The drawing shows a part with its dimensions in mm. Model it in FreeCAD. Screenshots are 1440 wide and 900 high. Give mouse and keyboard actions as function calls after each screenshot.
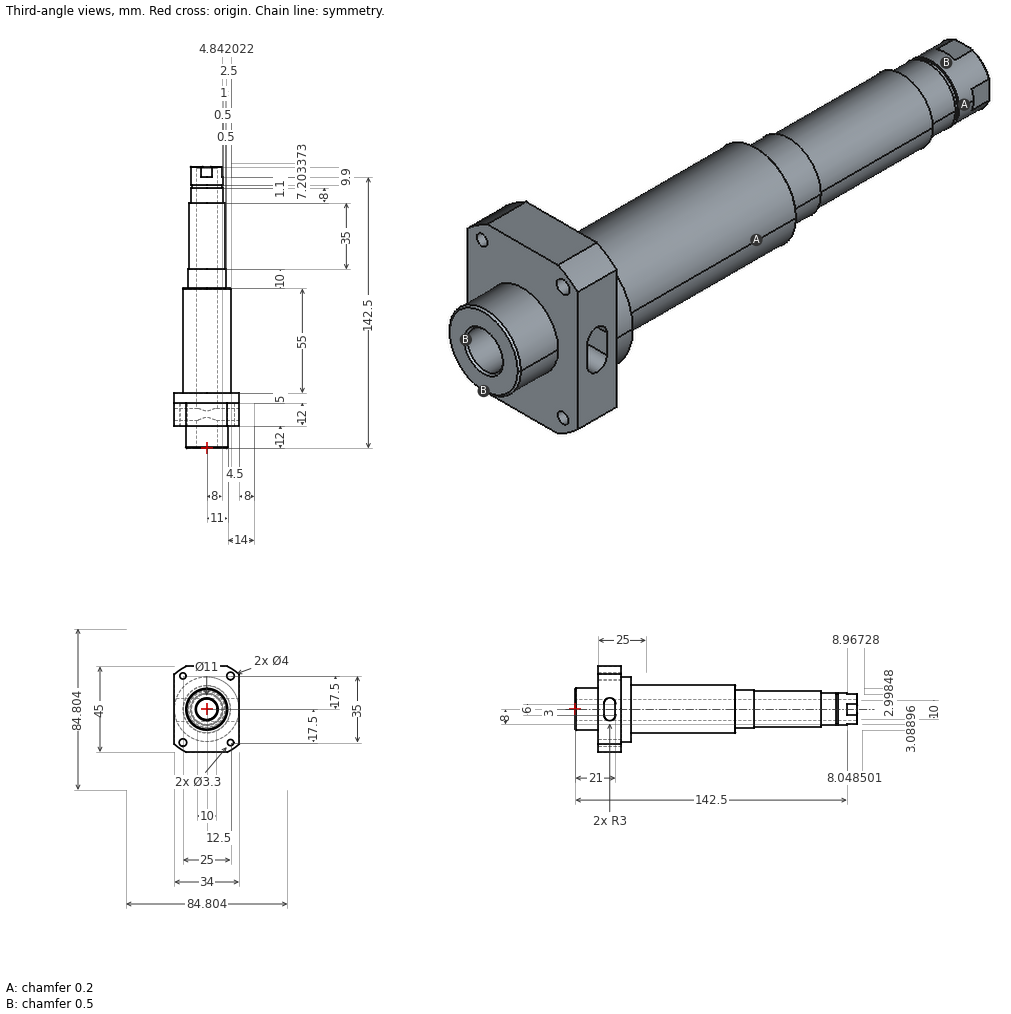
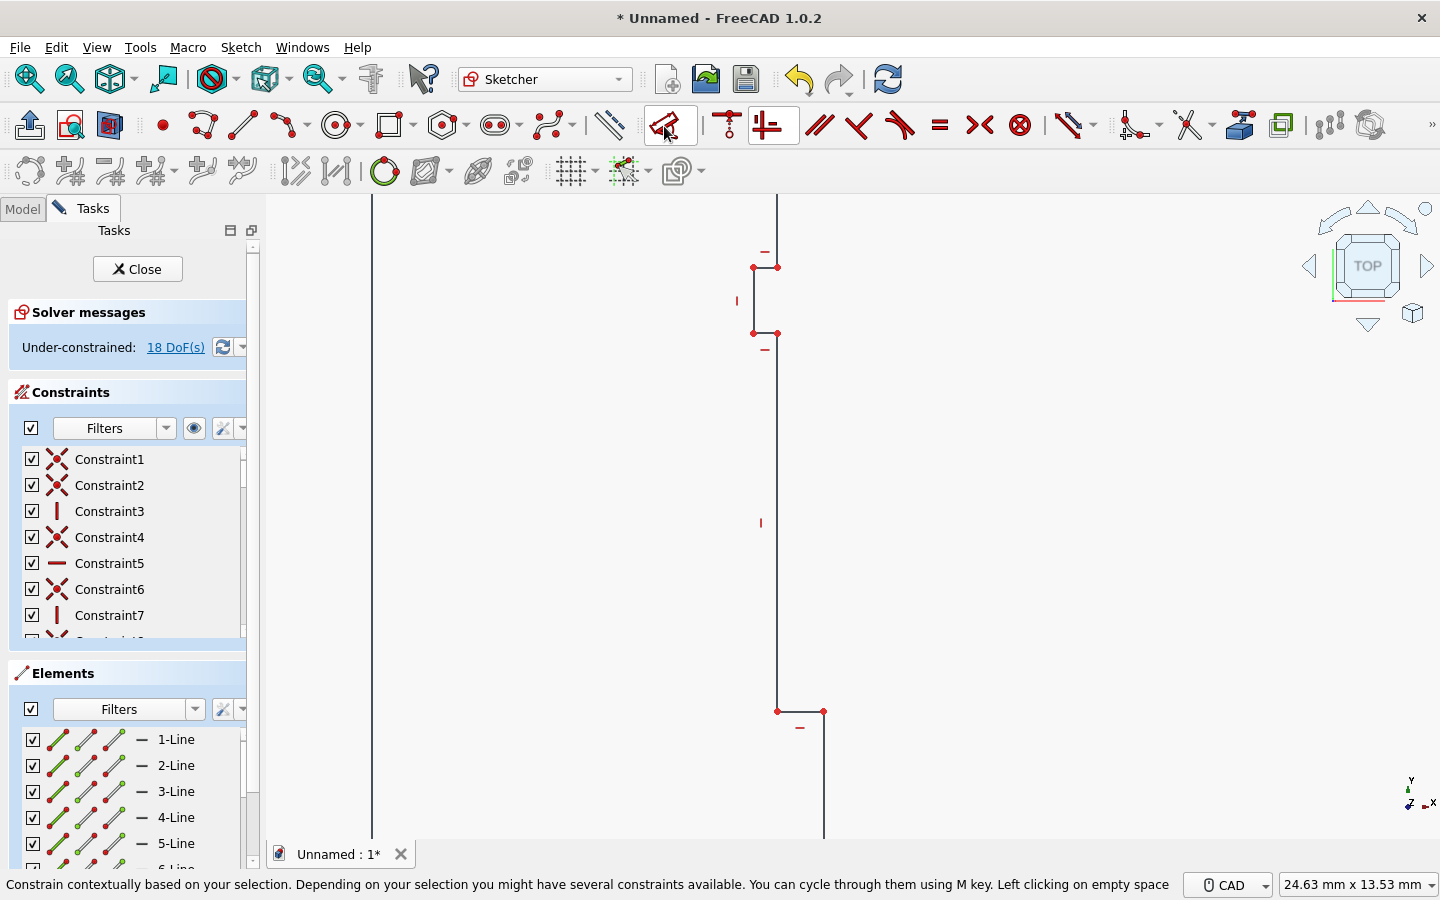
scroll(773, 335, down, 14)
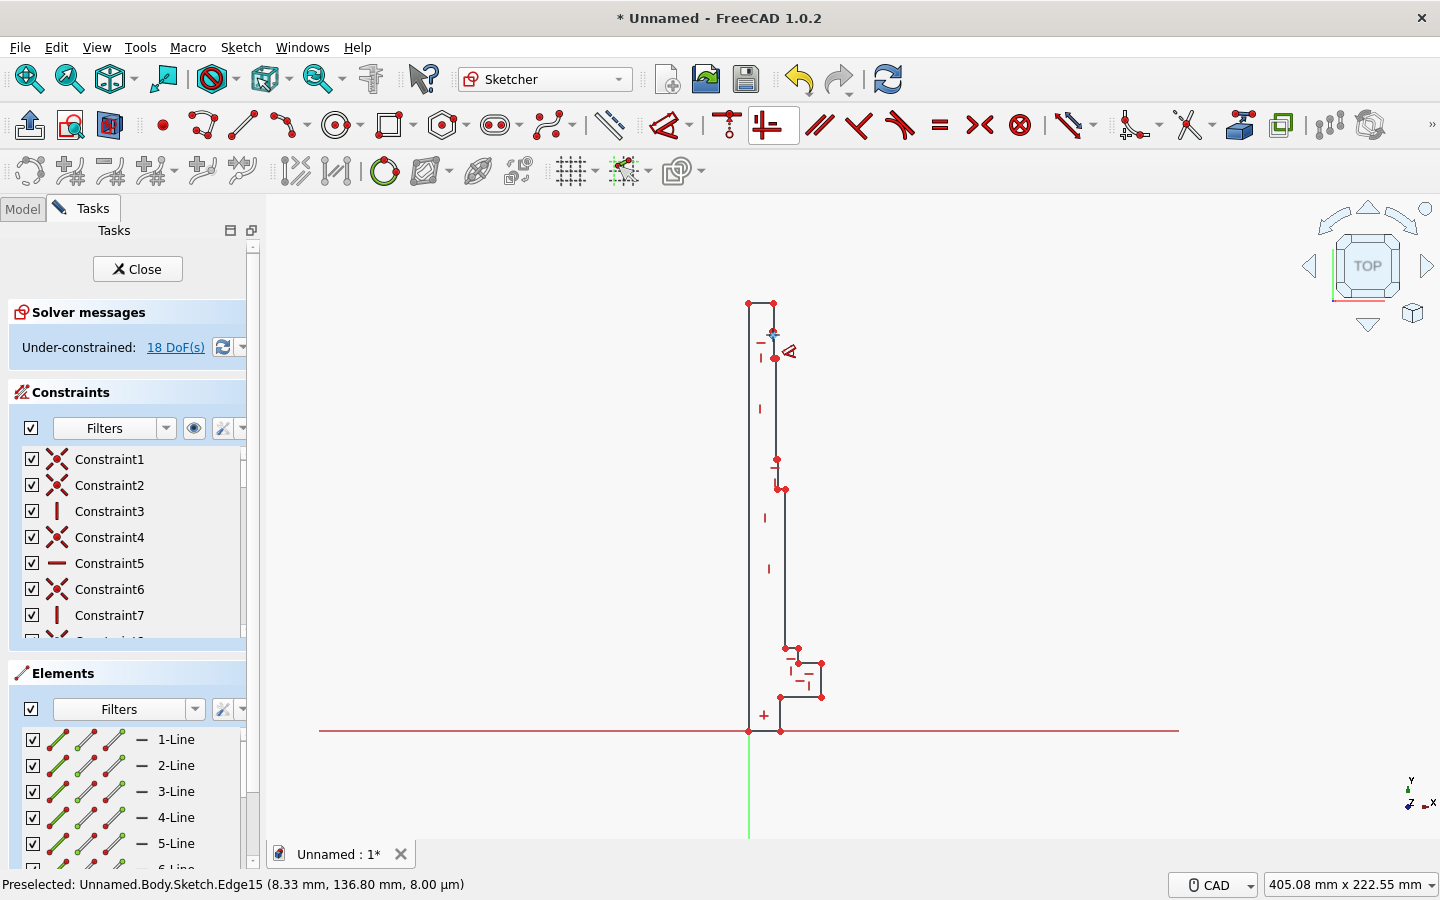
scroll(815, 663, up, 4)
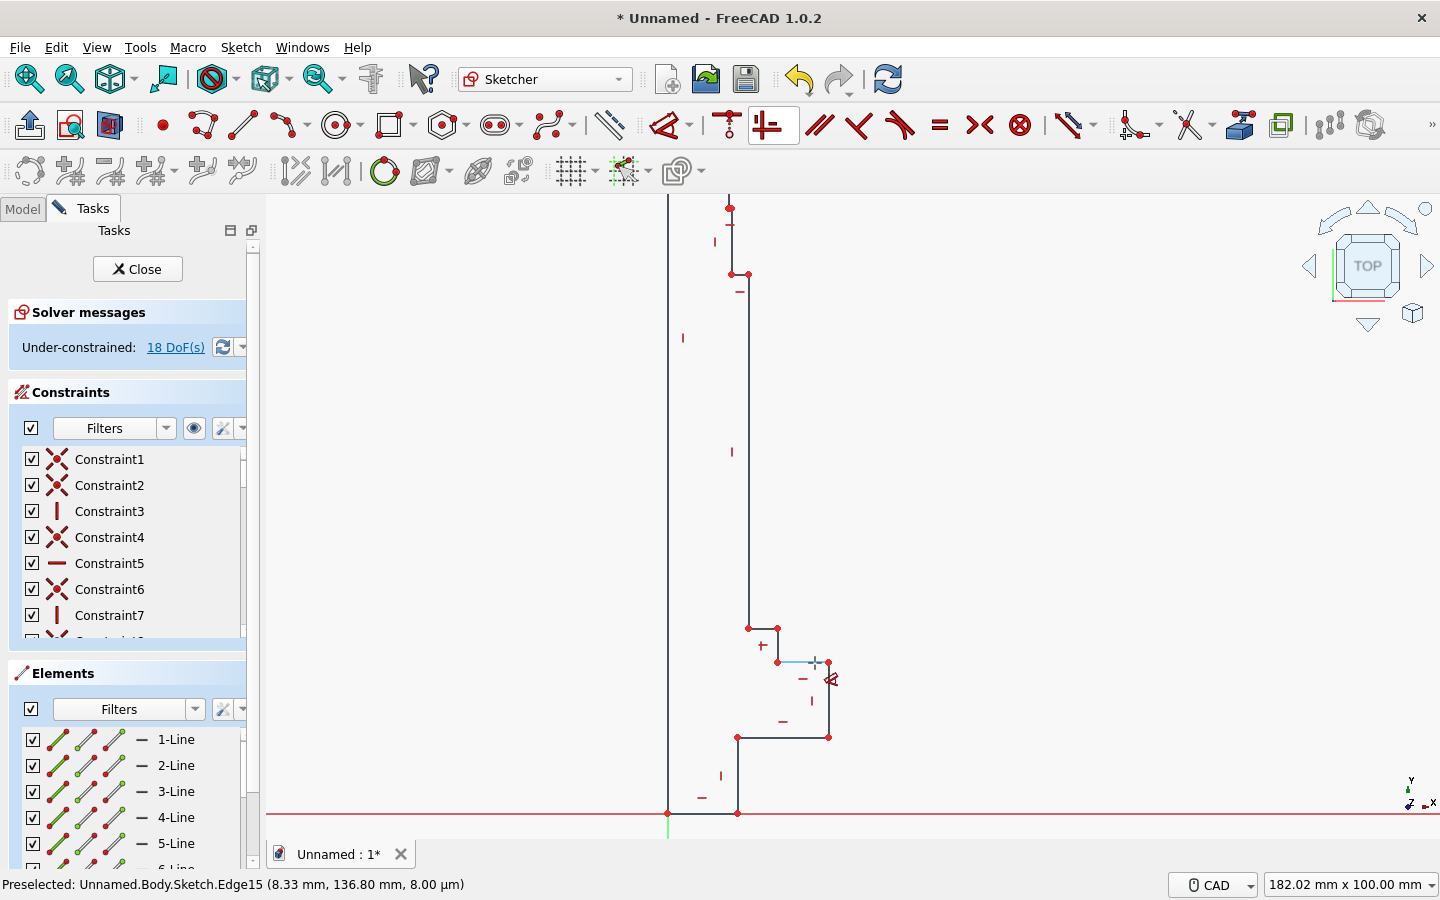
click(813, 662)
click(803, 696)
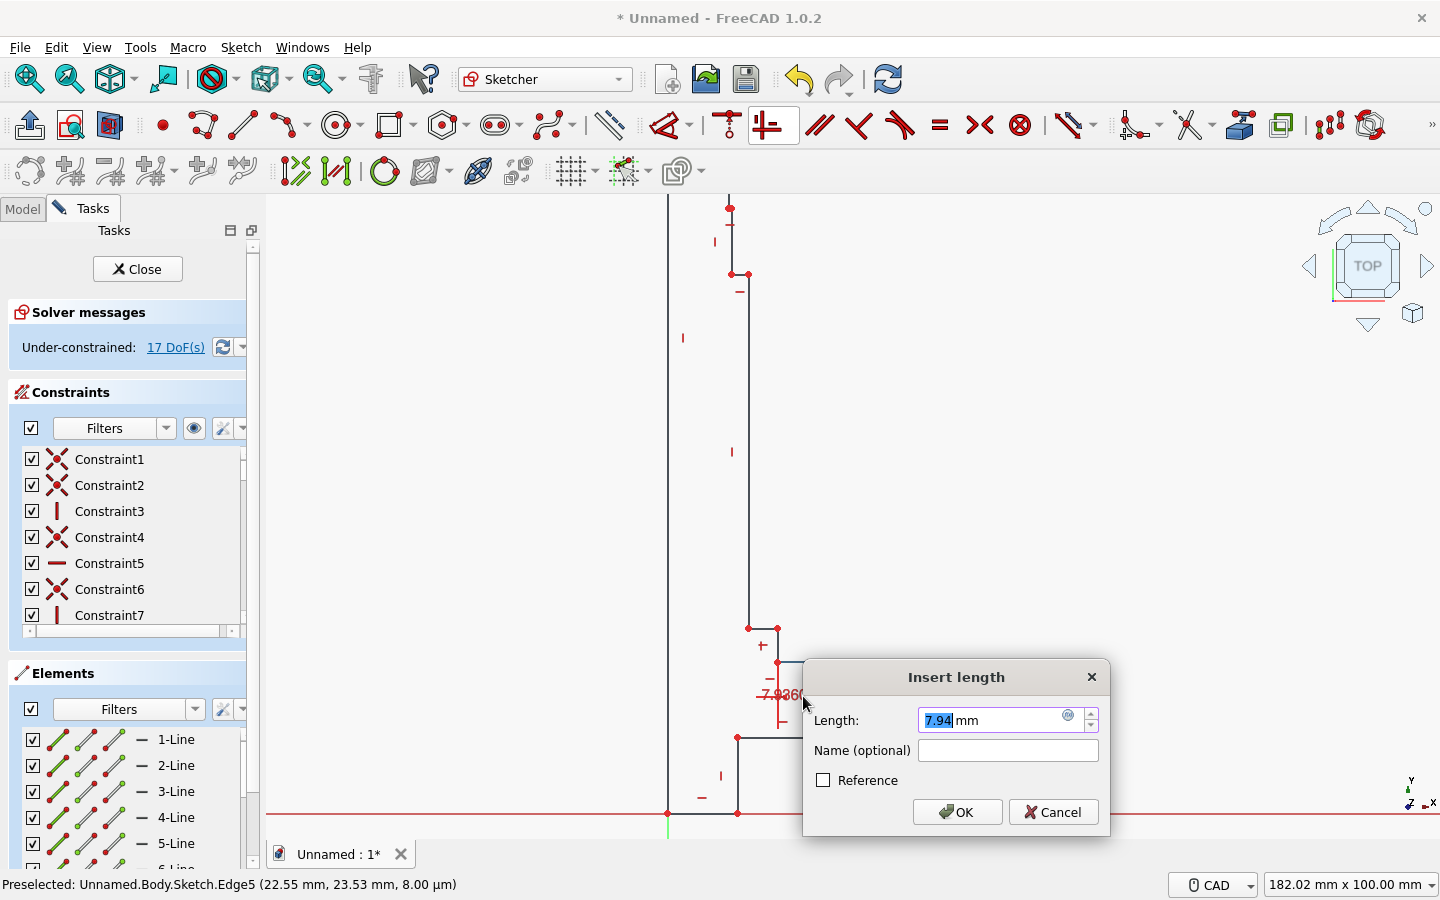
text(8)
key(Return)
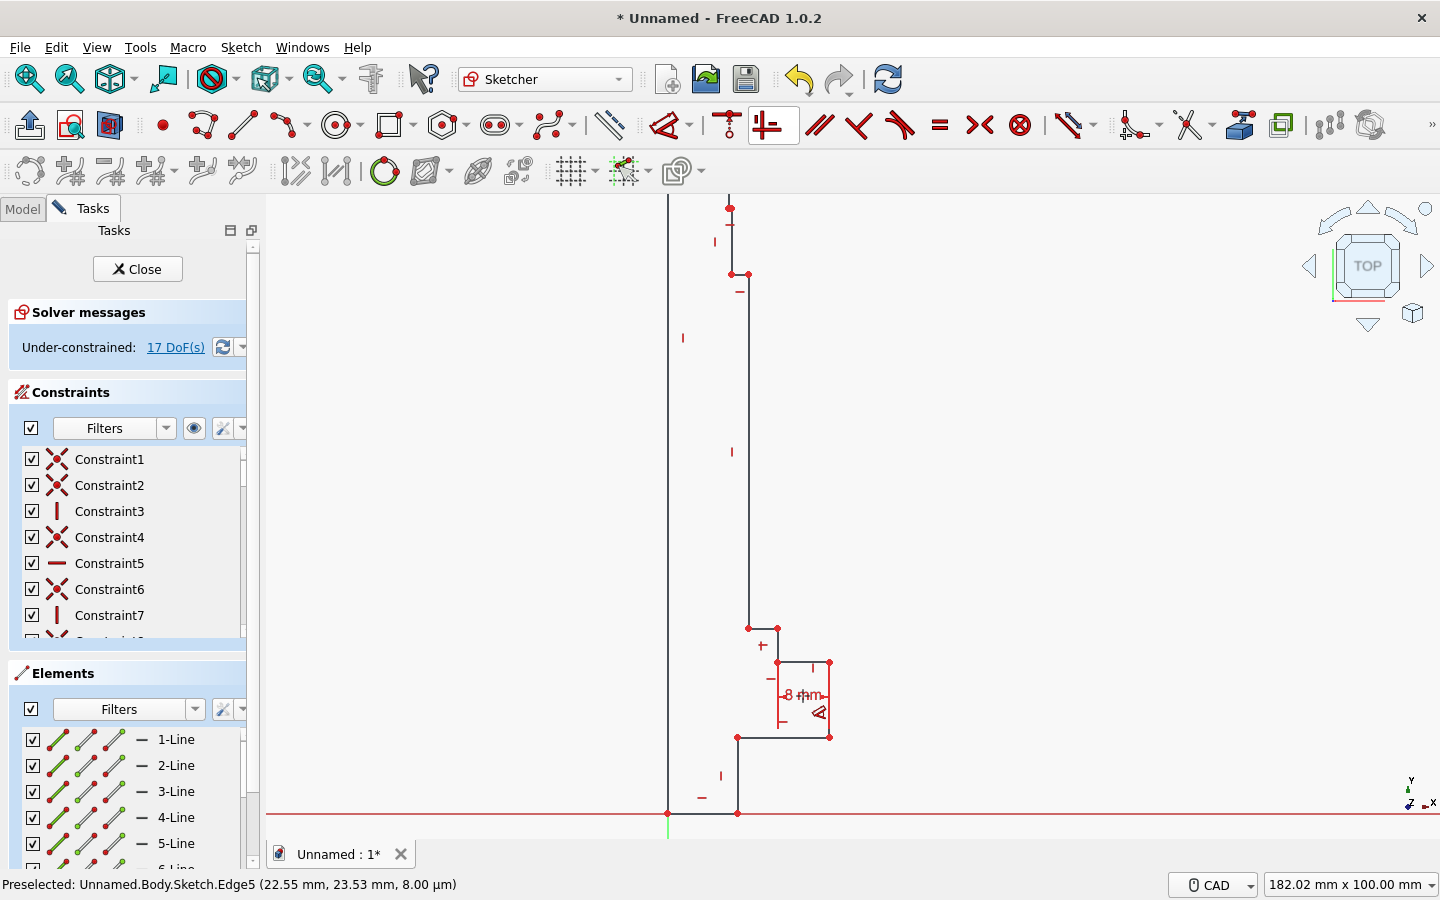
scroll(778, 652, up, 2)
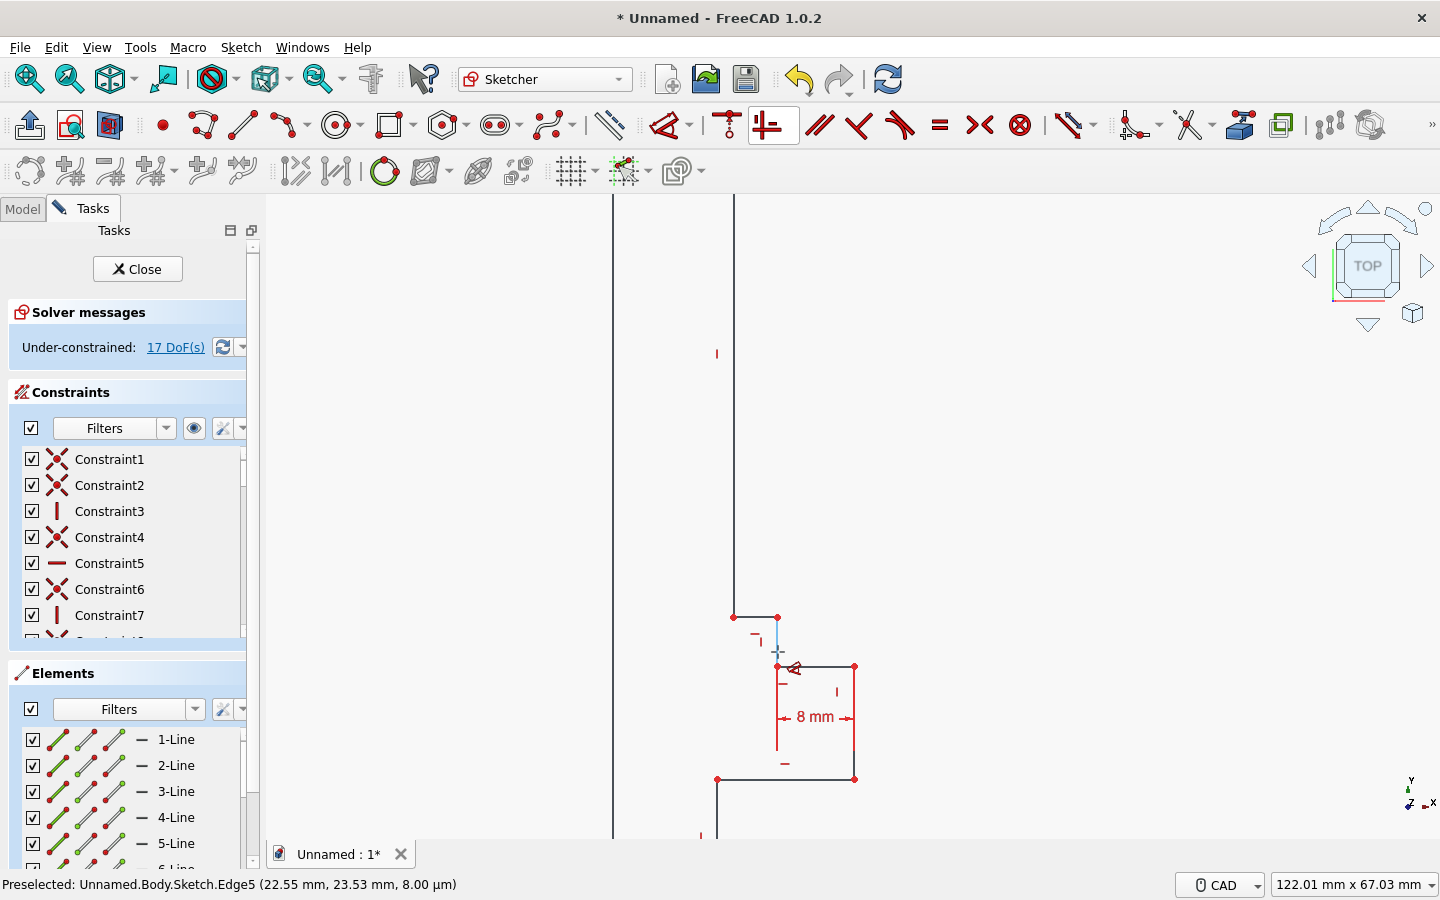
click(777, 652)
click(811, 642)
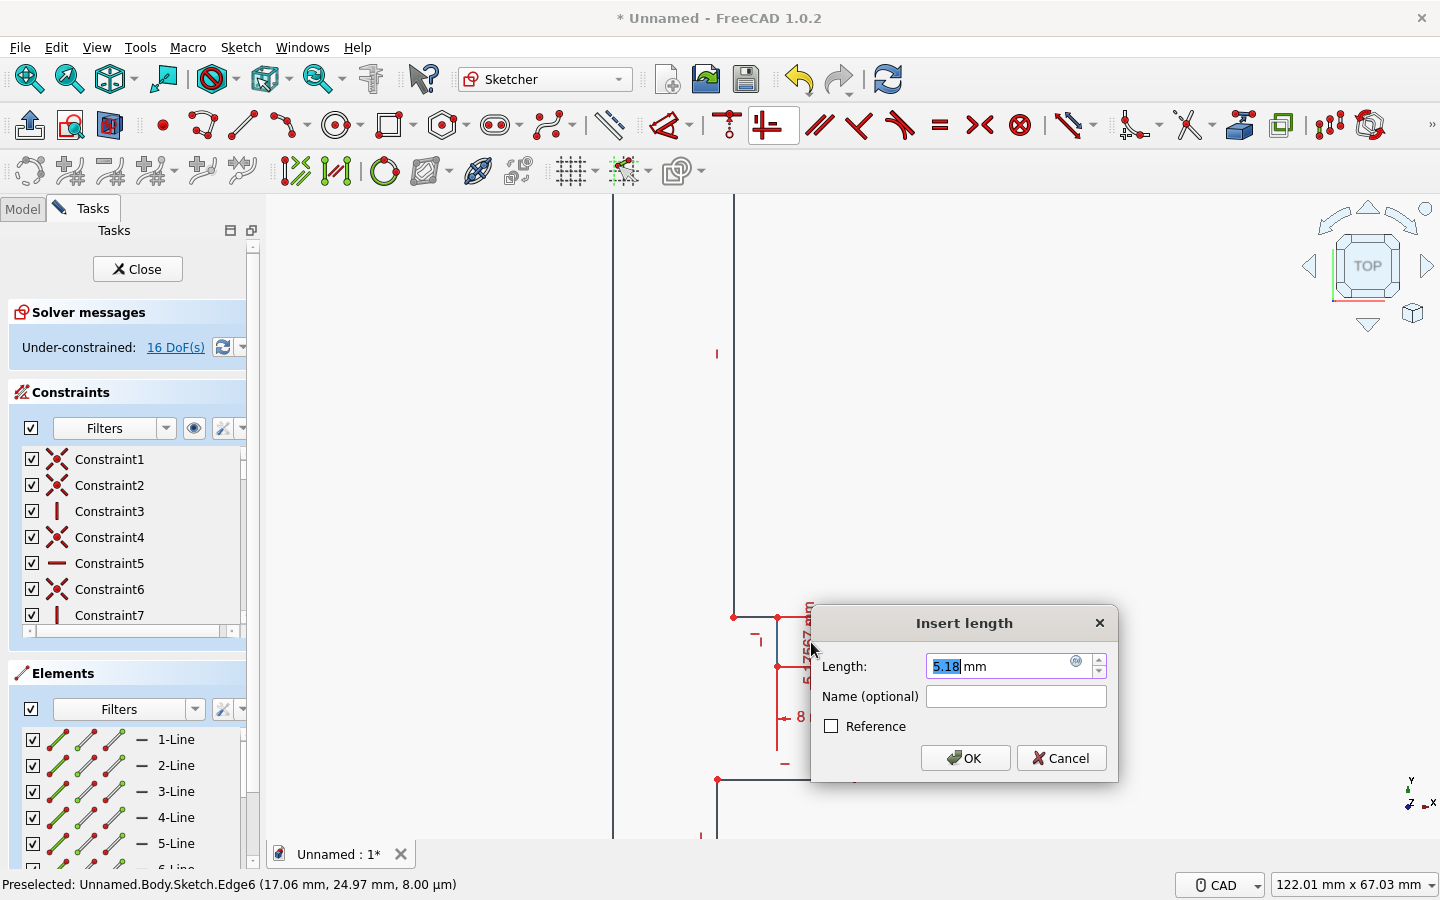
text(5)
key(Return)